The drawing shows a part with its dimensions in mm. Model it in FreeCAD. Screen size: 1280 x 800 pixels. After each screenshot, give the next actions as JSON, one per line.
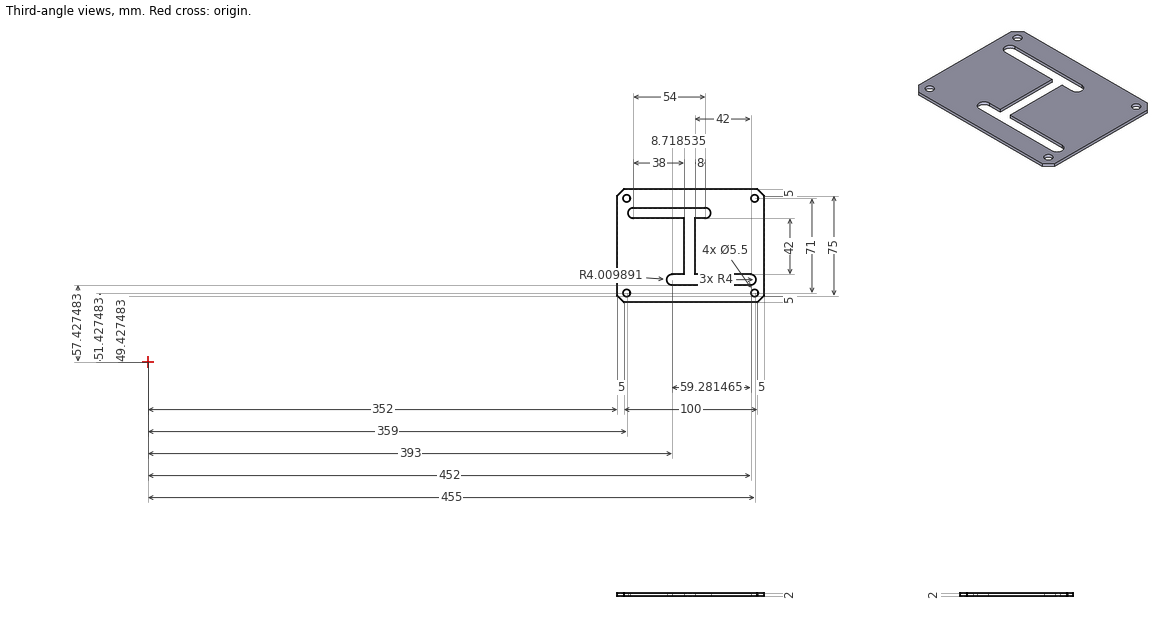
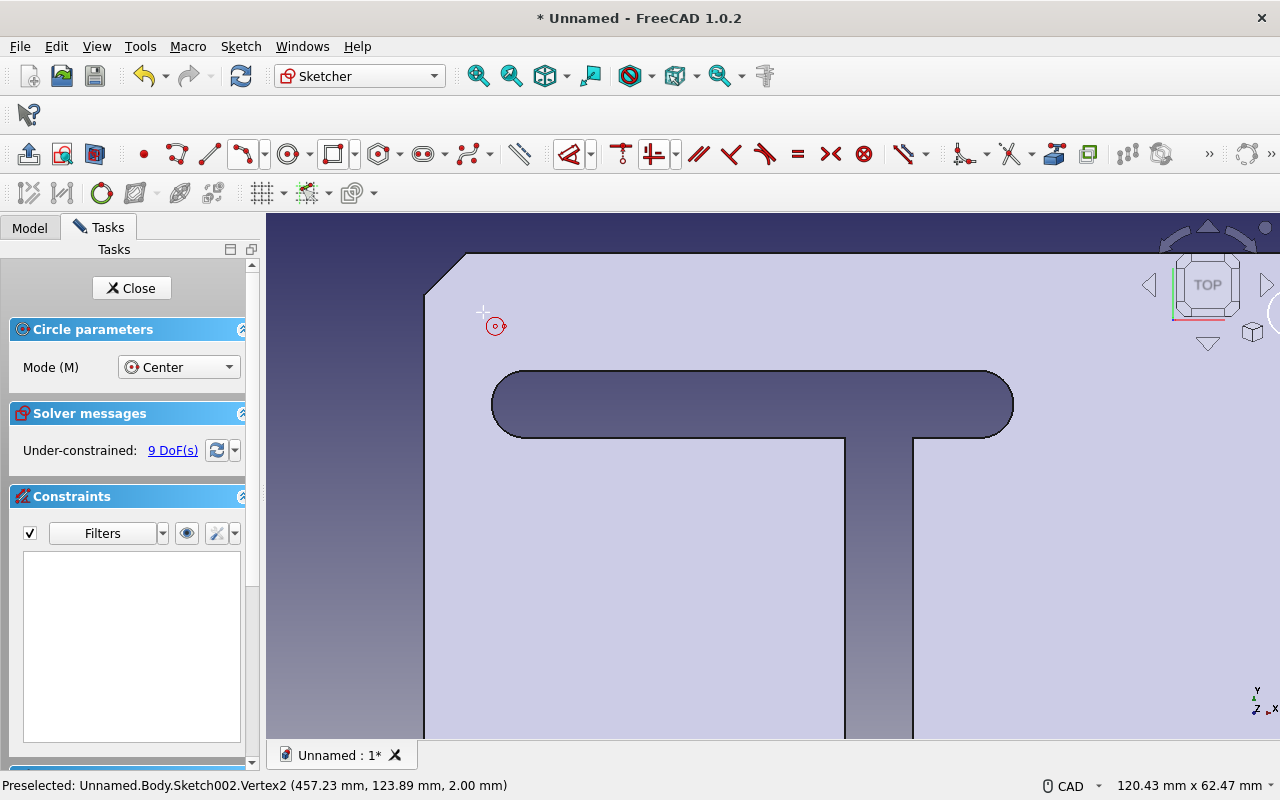
{"action": "left_click", "coordinate": [483, 312]}
{"action": "left_click", "coordinate": [500, 295]}
{"action": "key", "text": "Escape"}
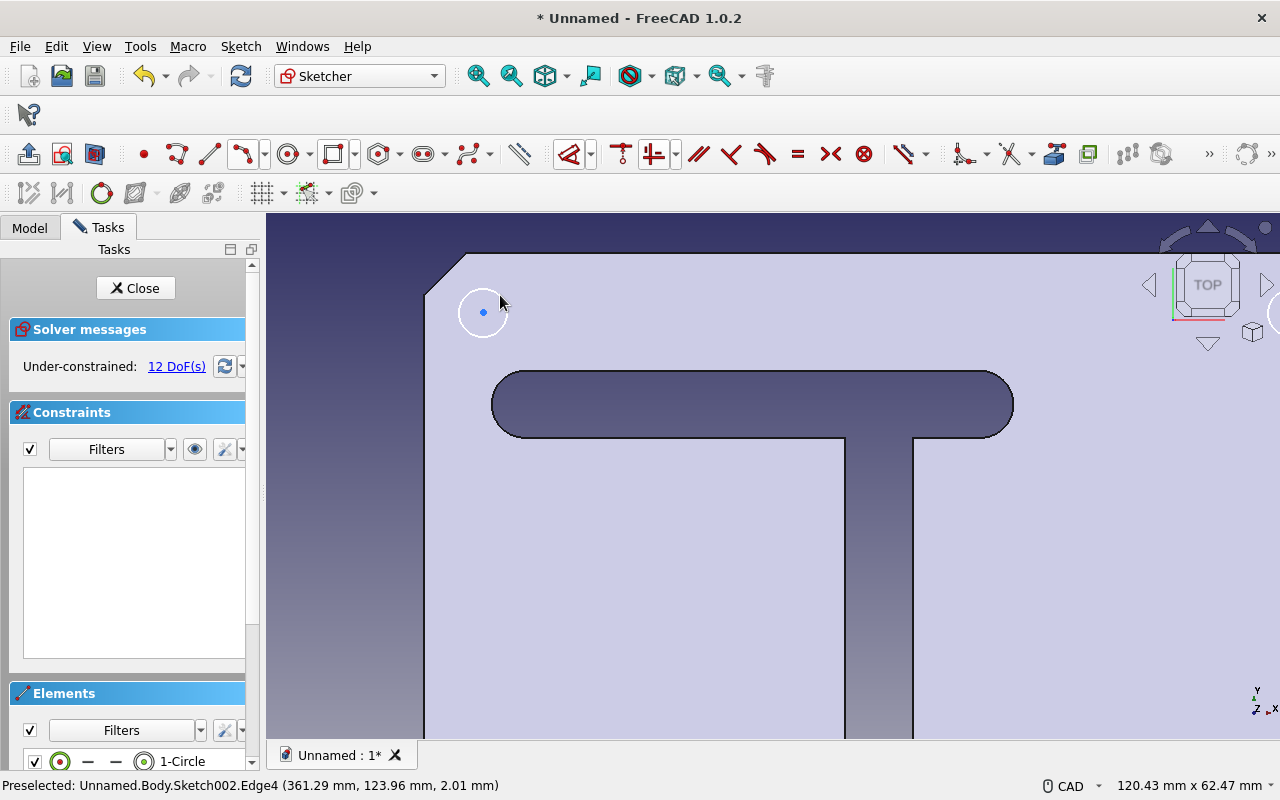
{"action": "scroll", "coordinate": [482, 312], "scroll_direction": "down", "scroll_amount": 3}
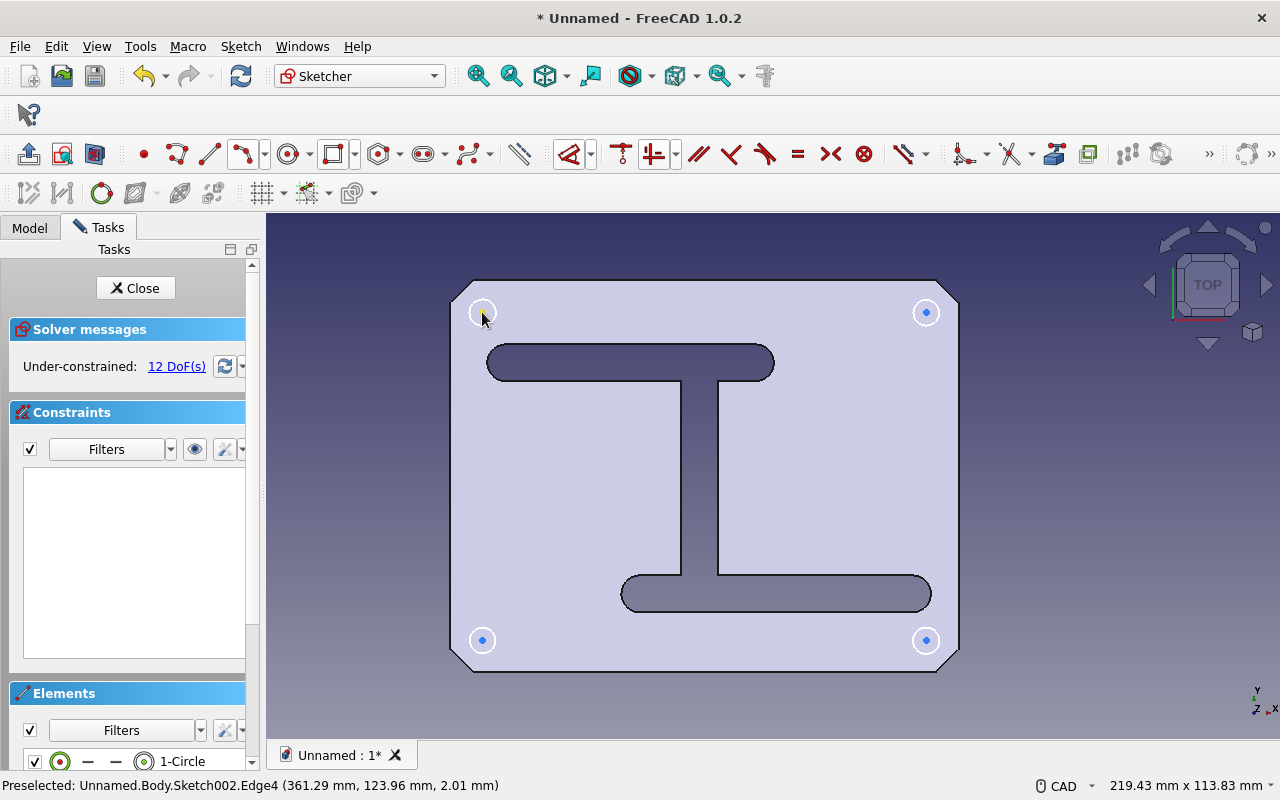
{"action": "left_click", "coordinate": [936, 631]}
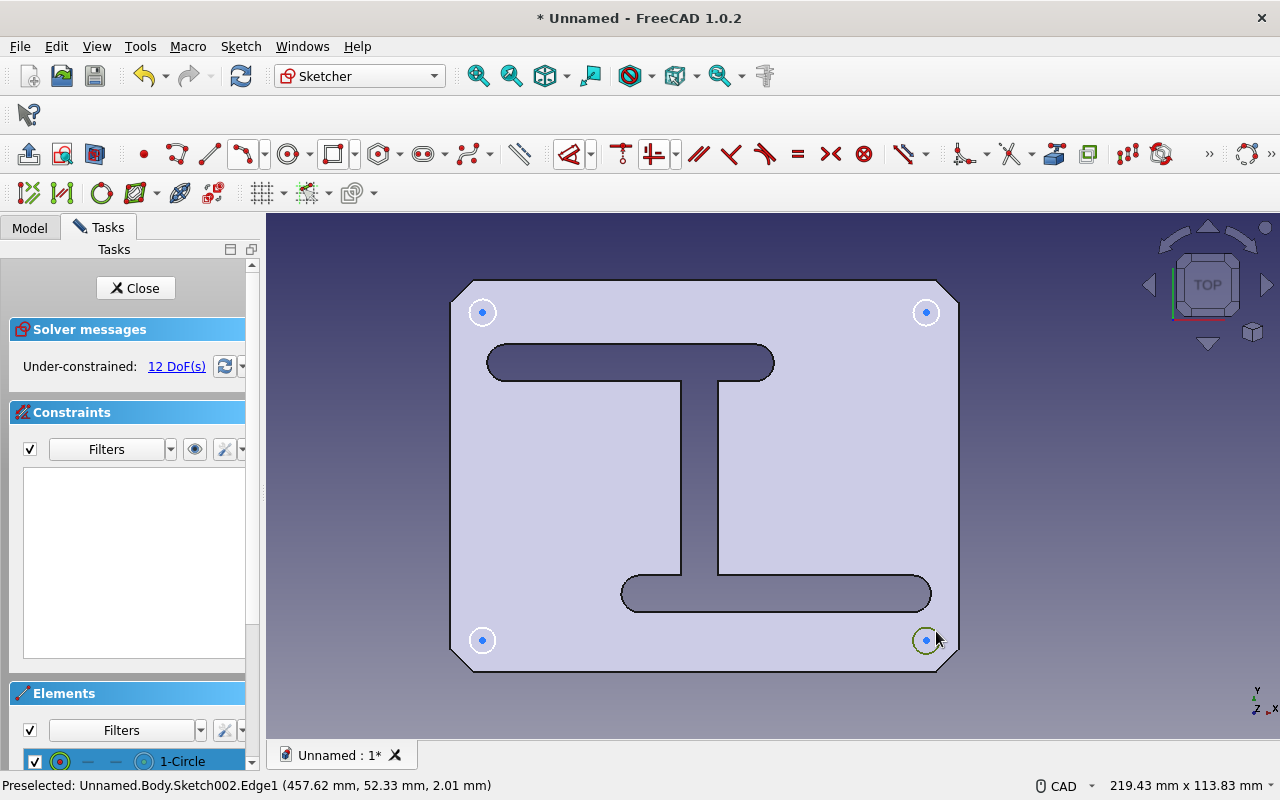
{"action": "left_click", "coordinate": [492, 631]}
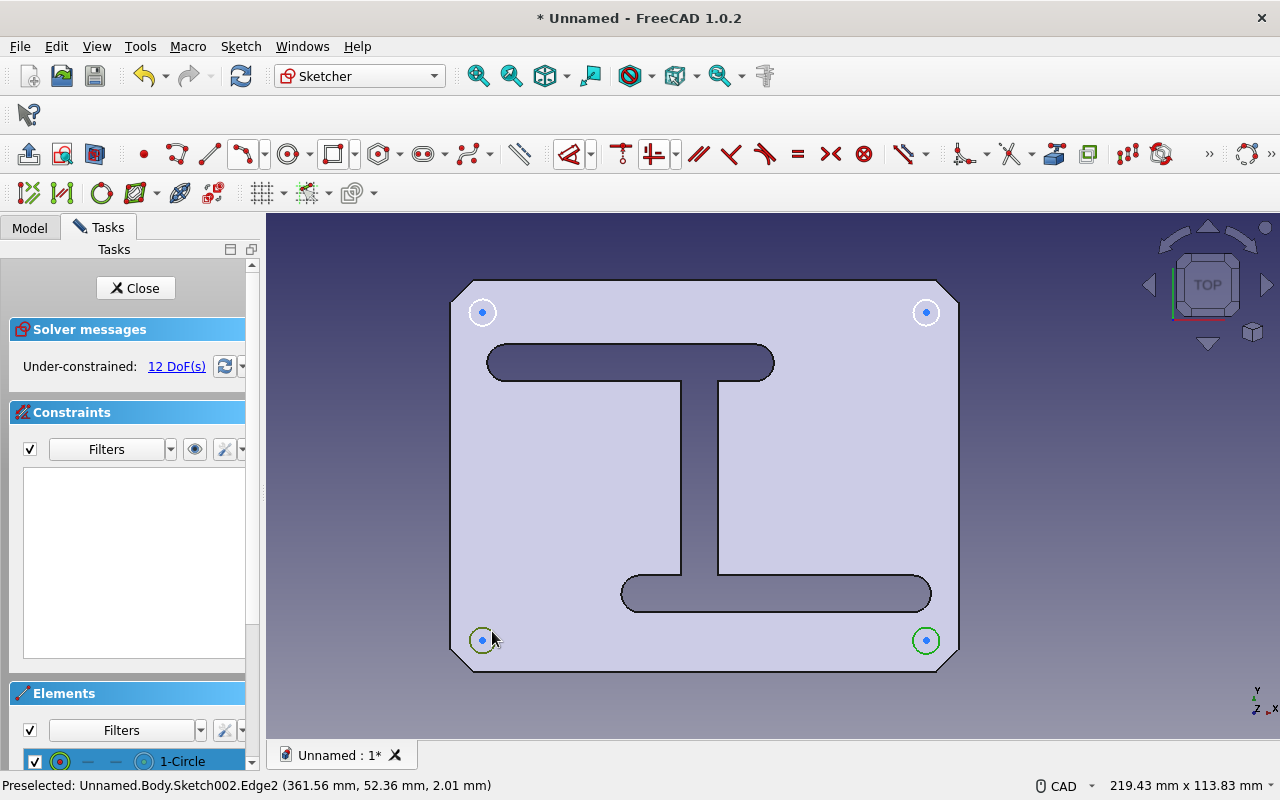
{"action": "left_click", "coordinate": [935, 304]}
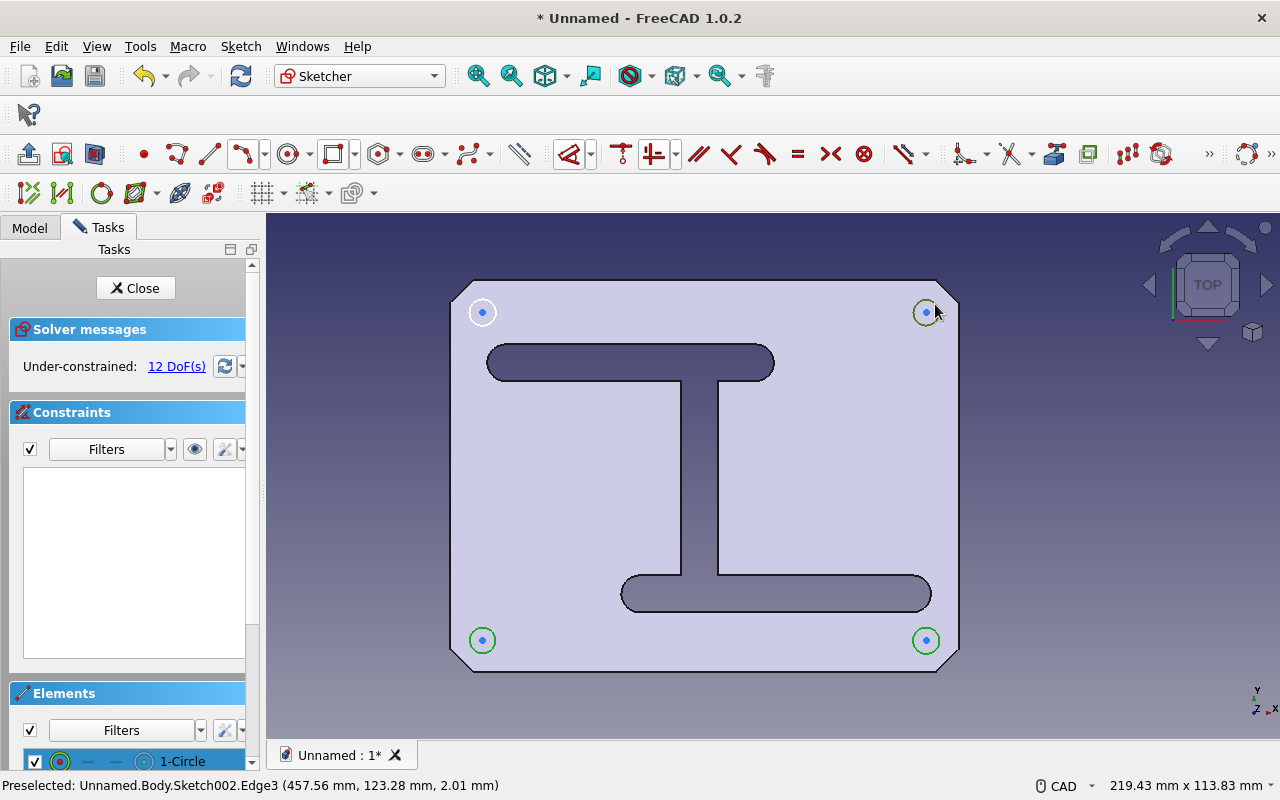
{"action": "left_click", "coordinate": [492, 303]}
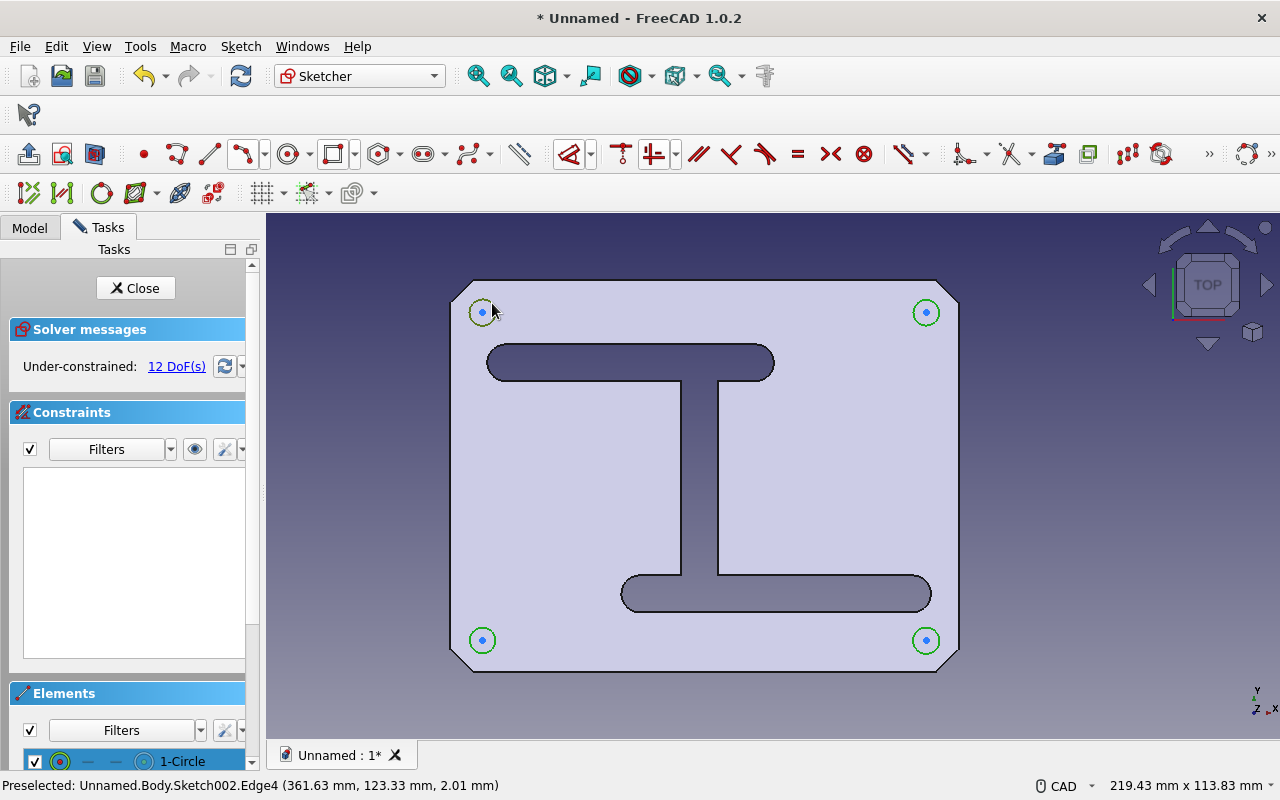
{"action": "key", "text": "e"}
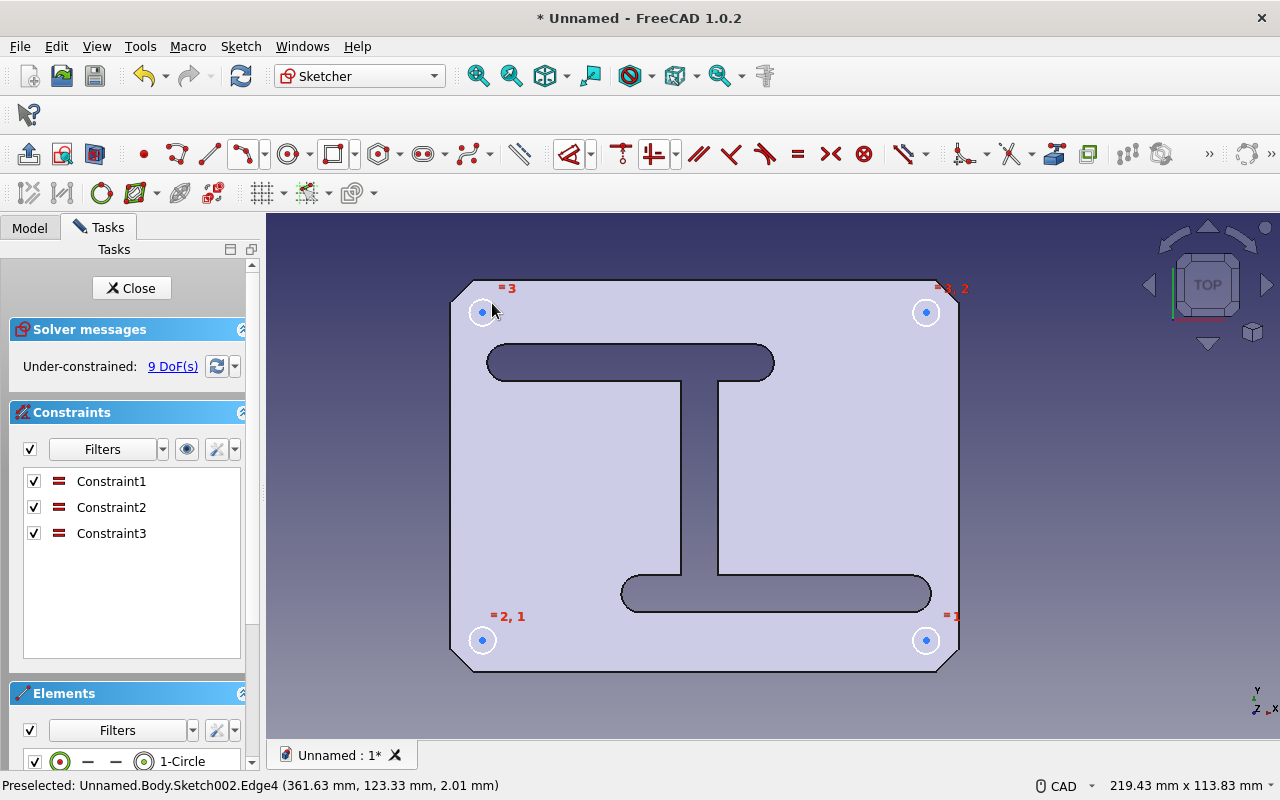
{"action": "left_click", "coordinate": [926, 641]}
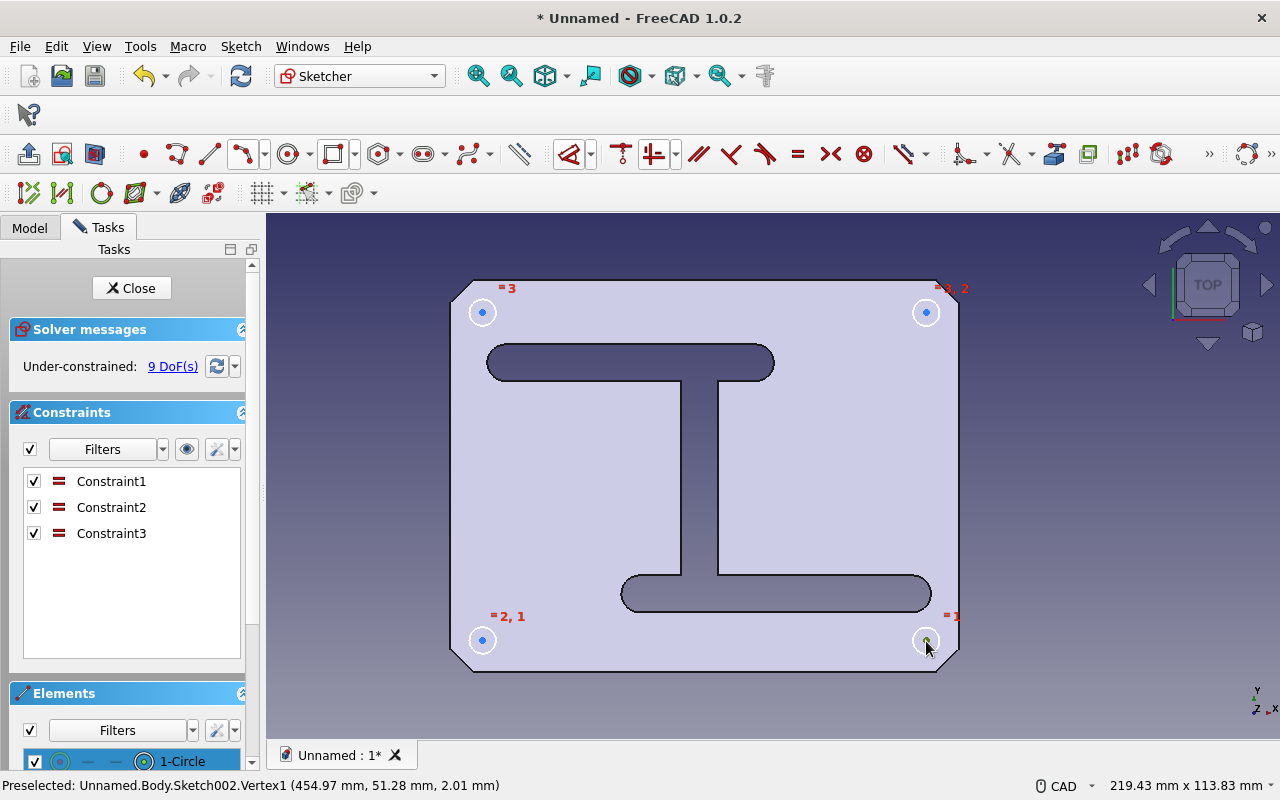
{"action": "left_click", "coordinate": [483, 640]}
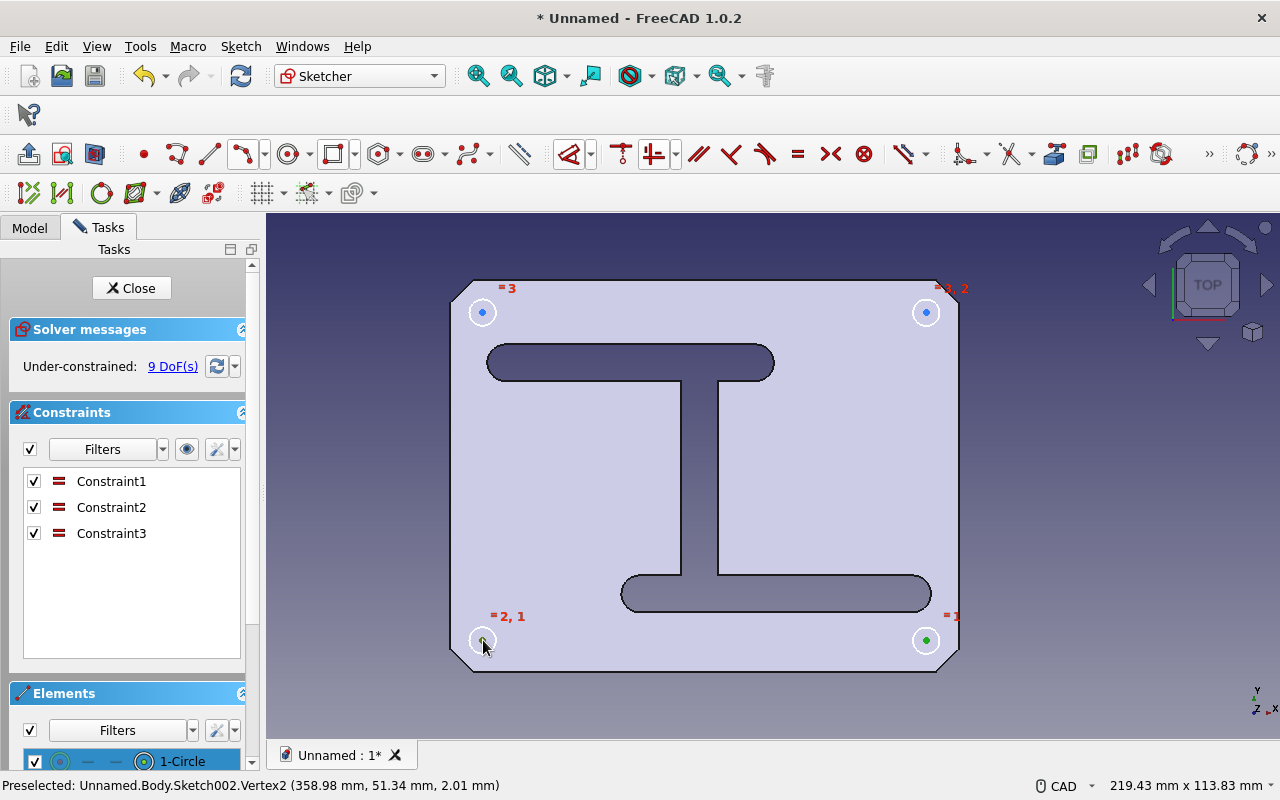
{"action": "left_click", "coordinate": [676, 154]}